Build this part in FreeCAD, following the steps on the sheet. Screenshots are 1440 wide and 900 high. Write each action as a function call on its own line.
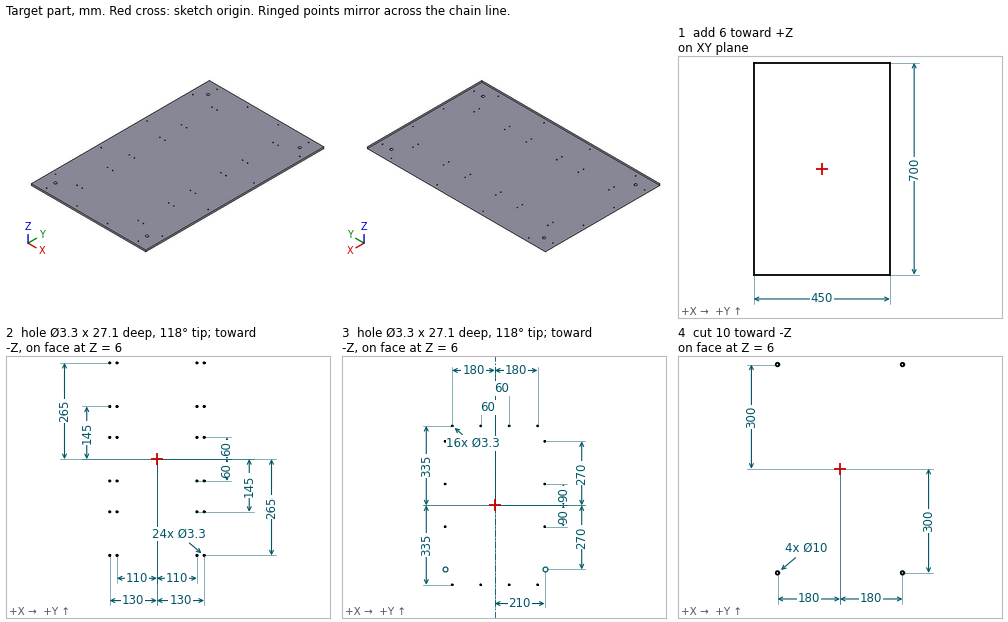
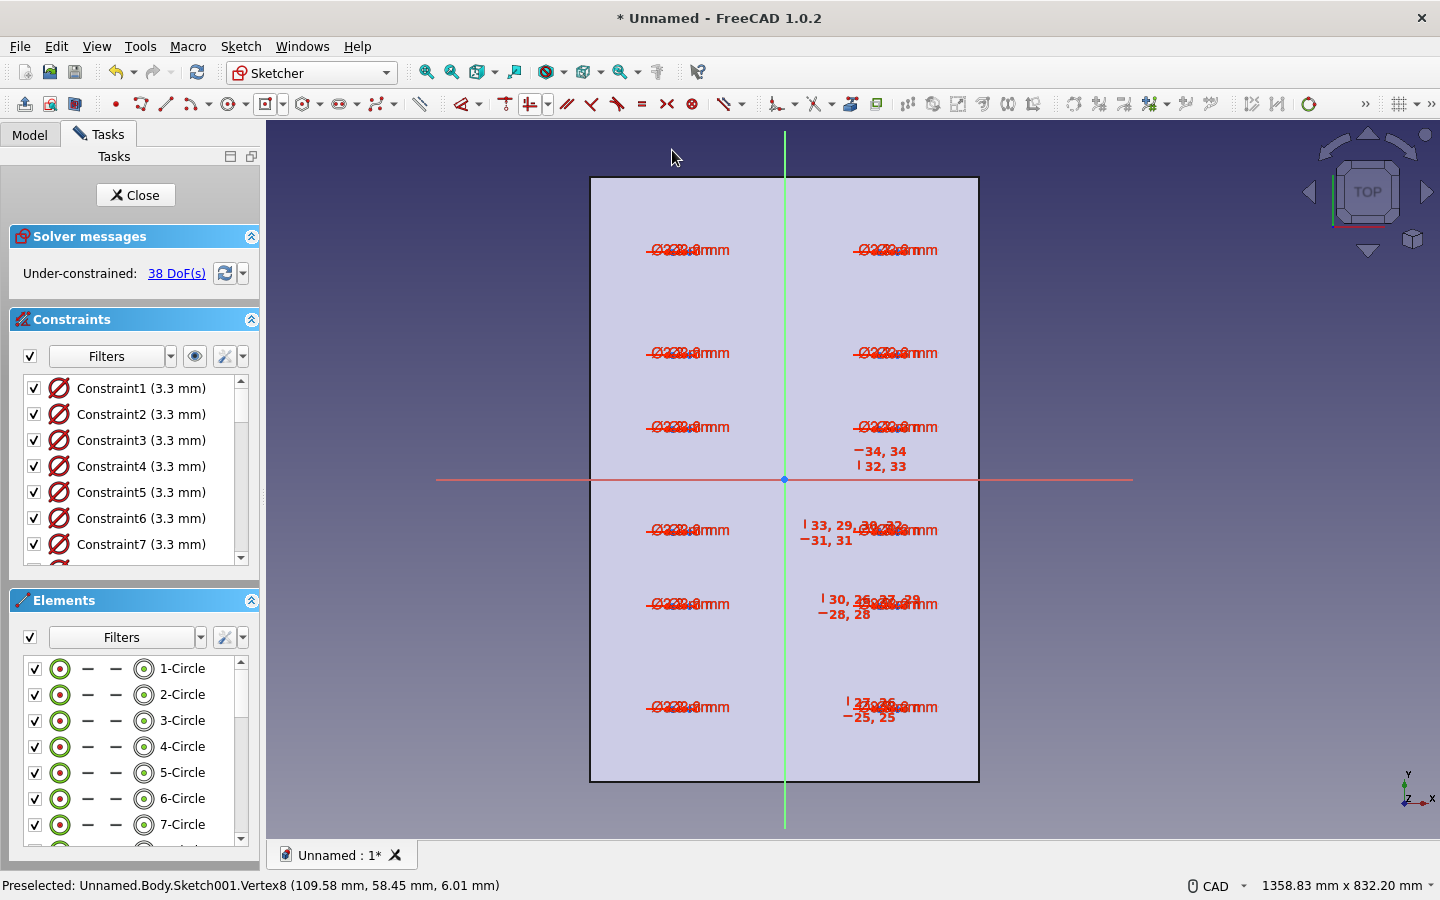
click(879, 709)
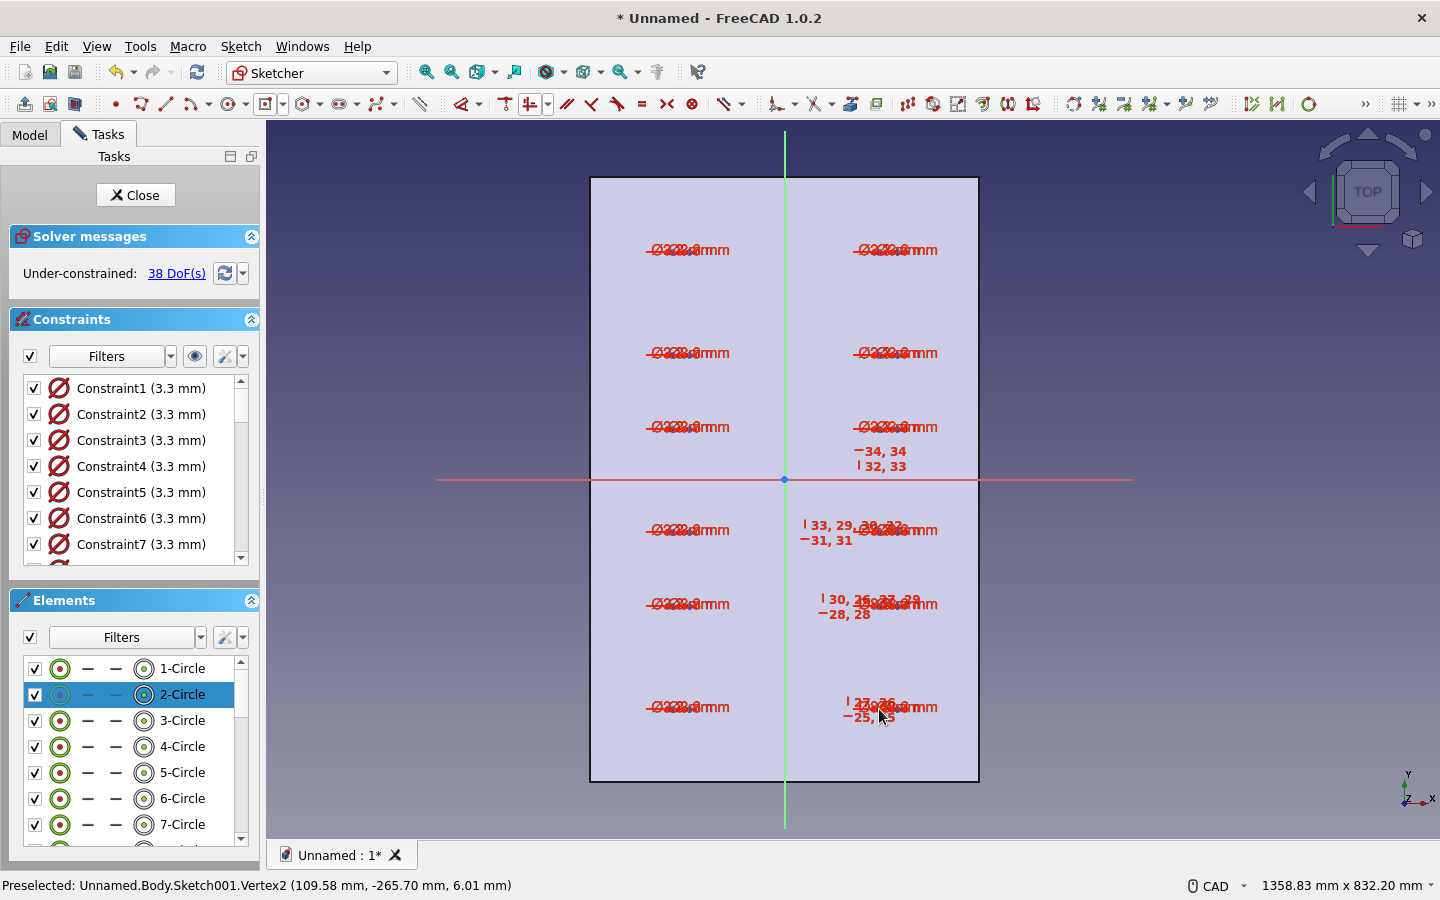
click(672, 709)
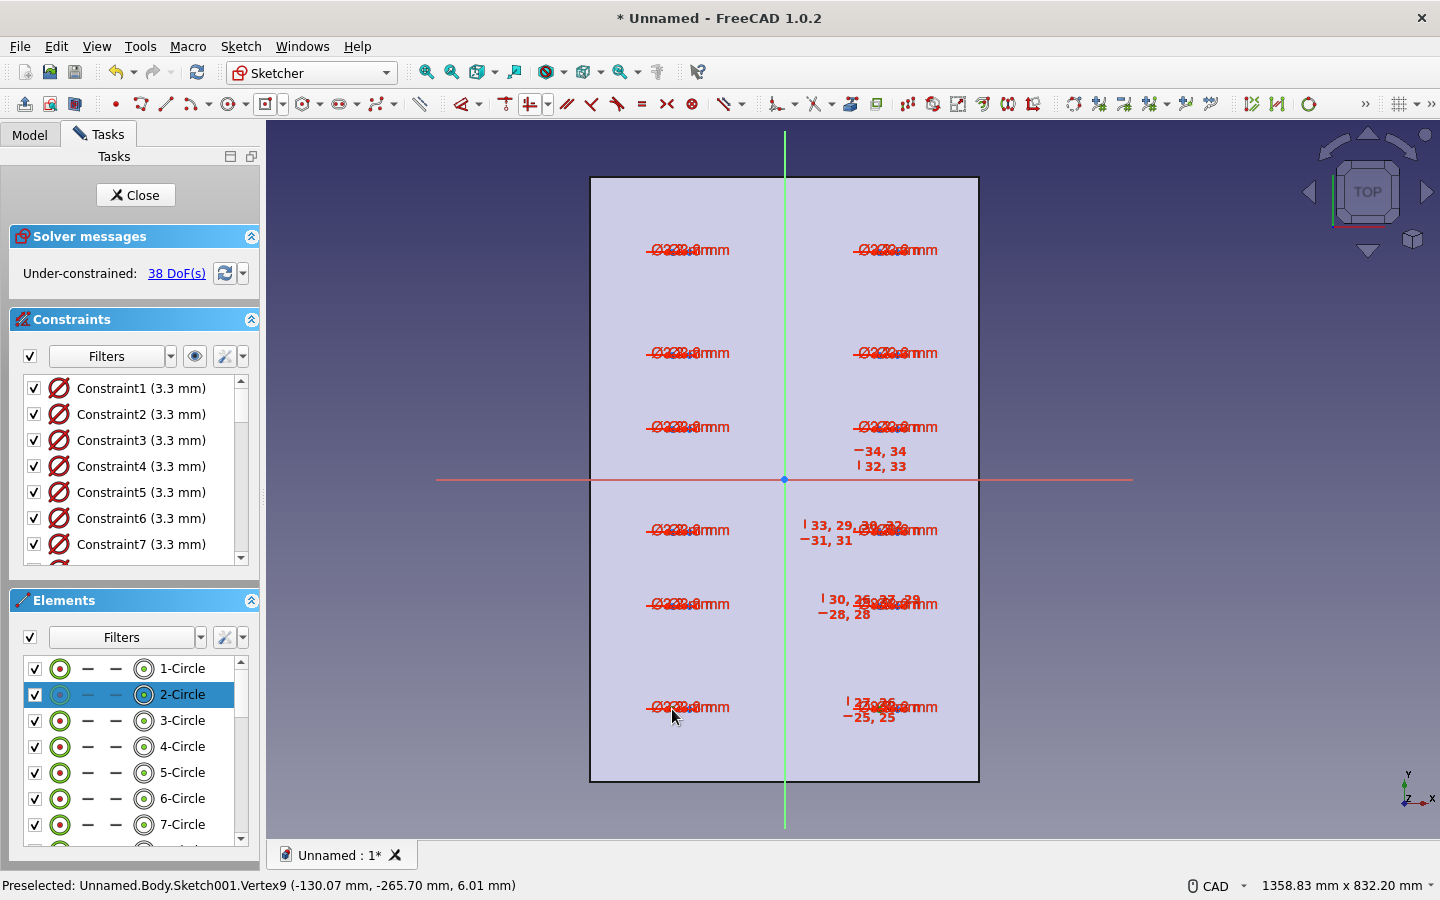
key(h)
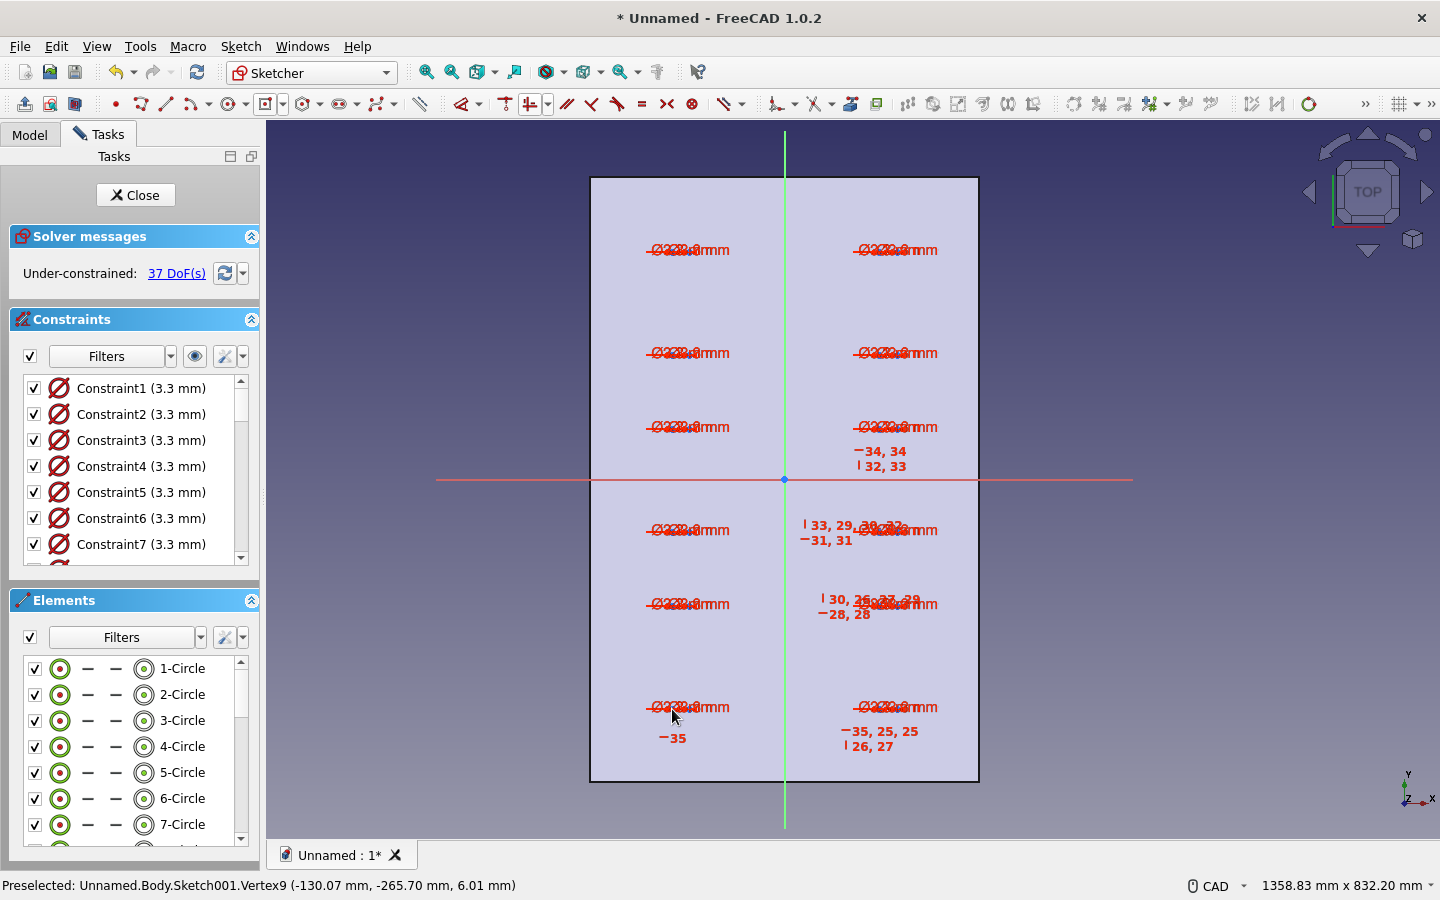
click(672, 709)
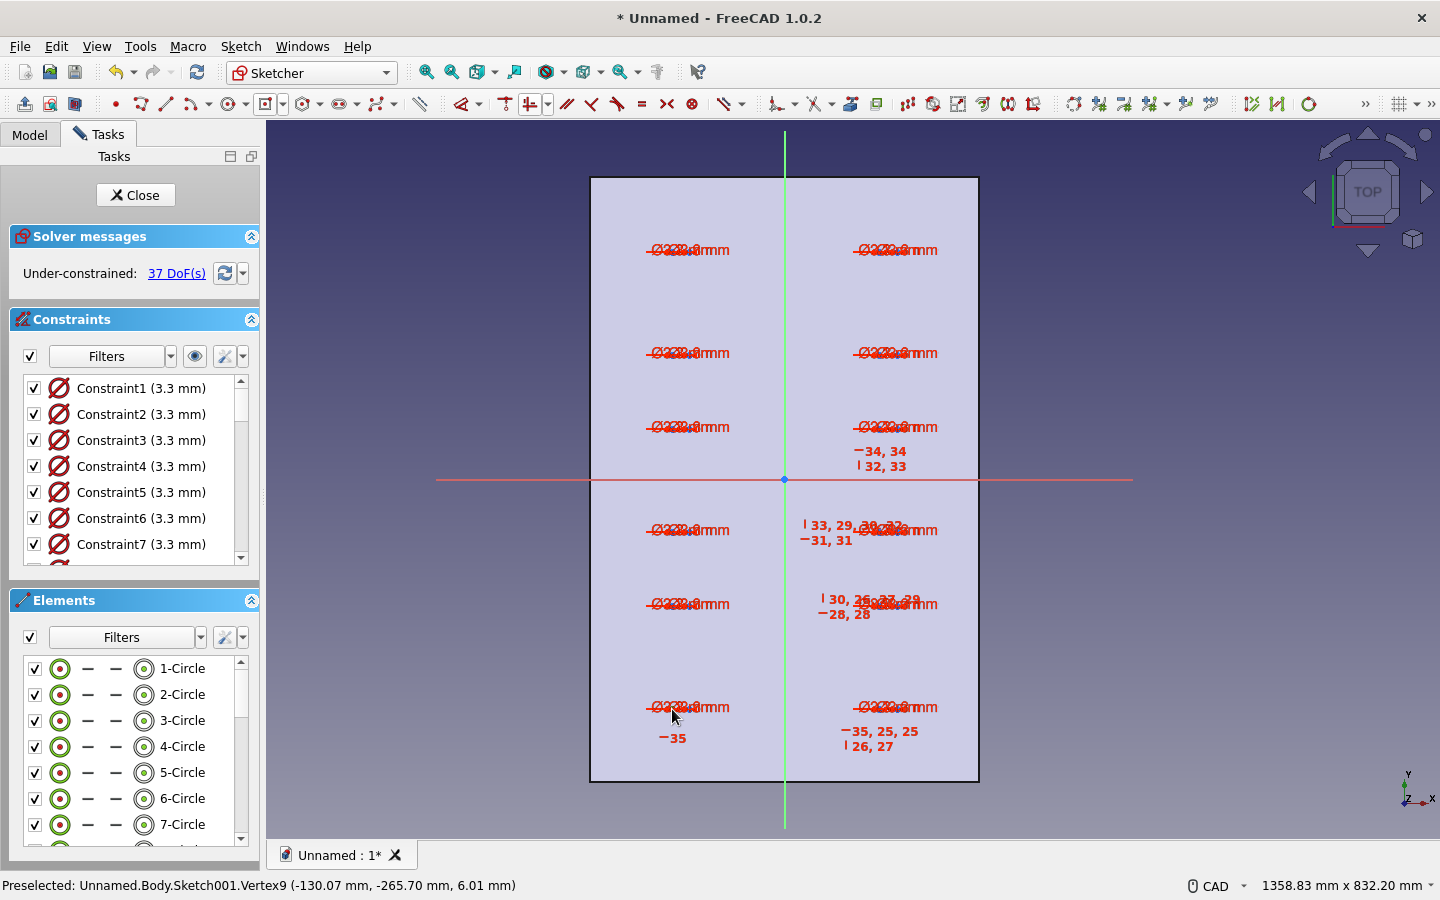
click(689, 709)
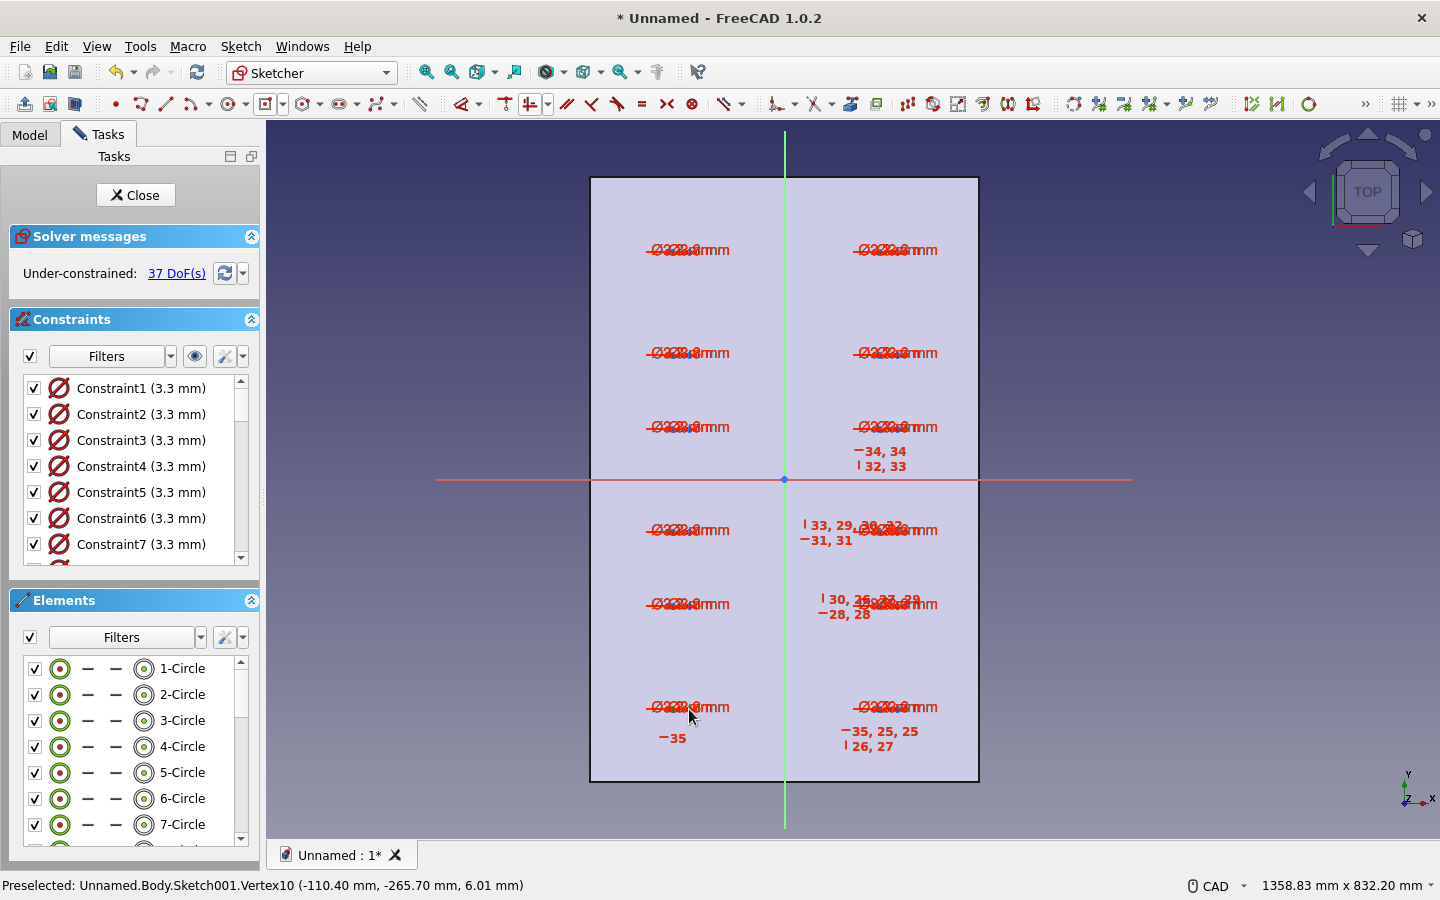
key(h)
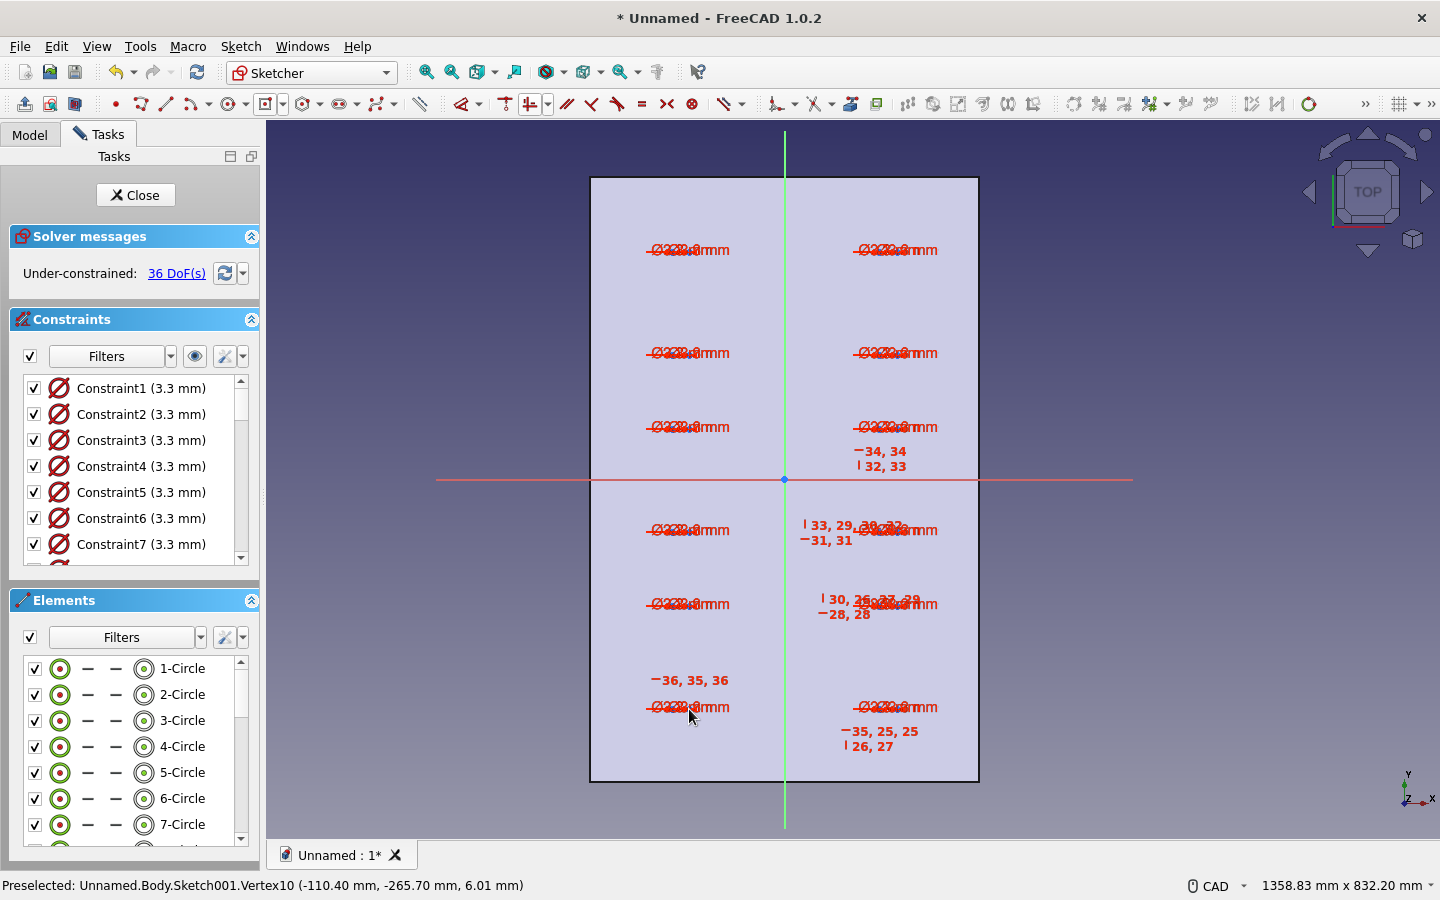
click(672, 709)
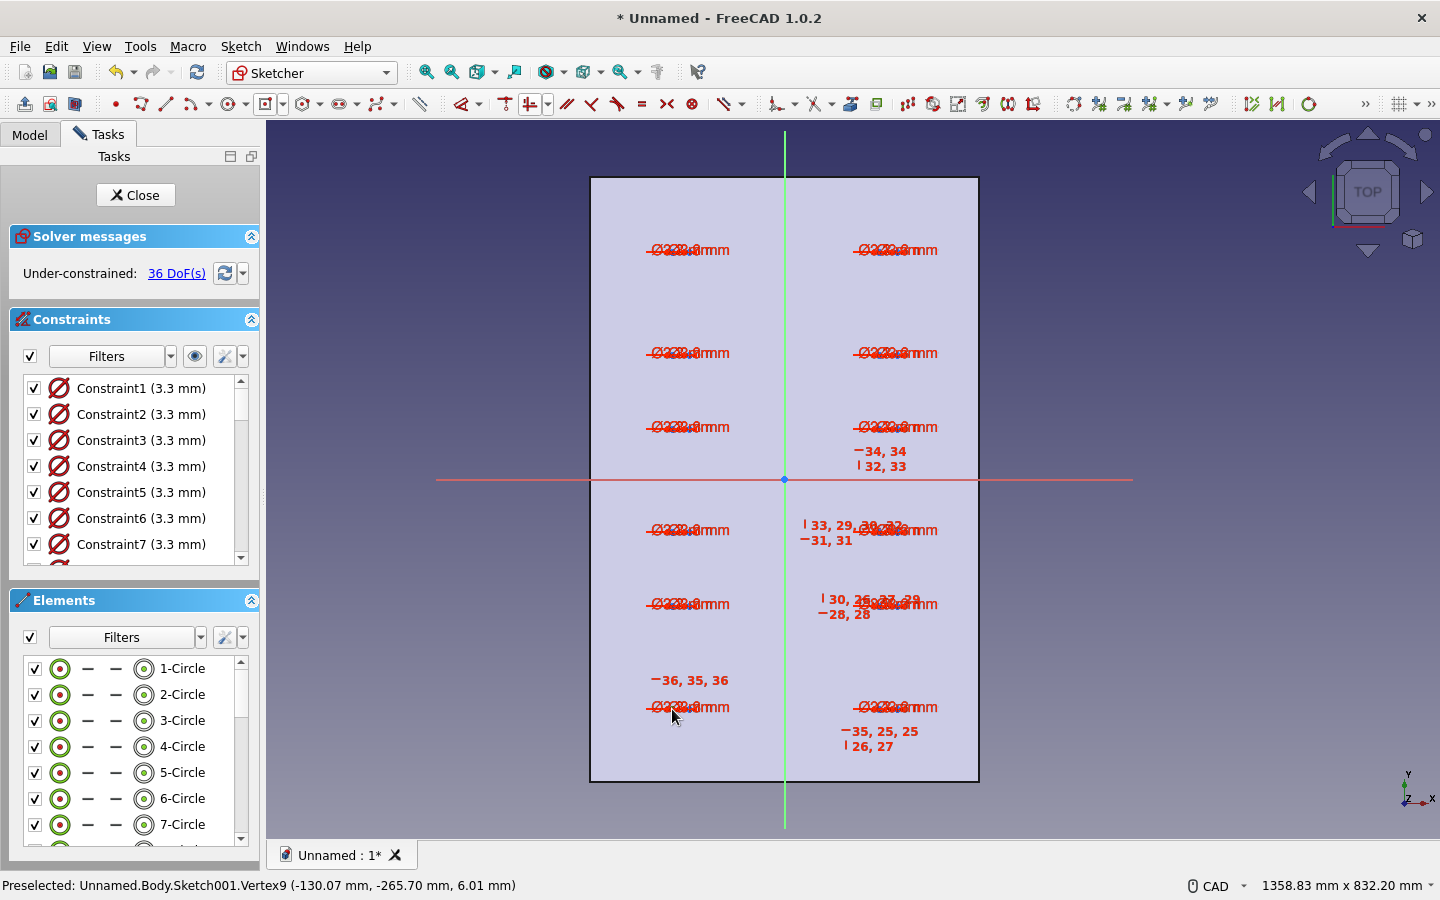
click(672, 606)